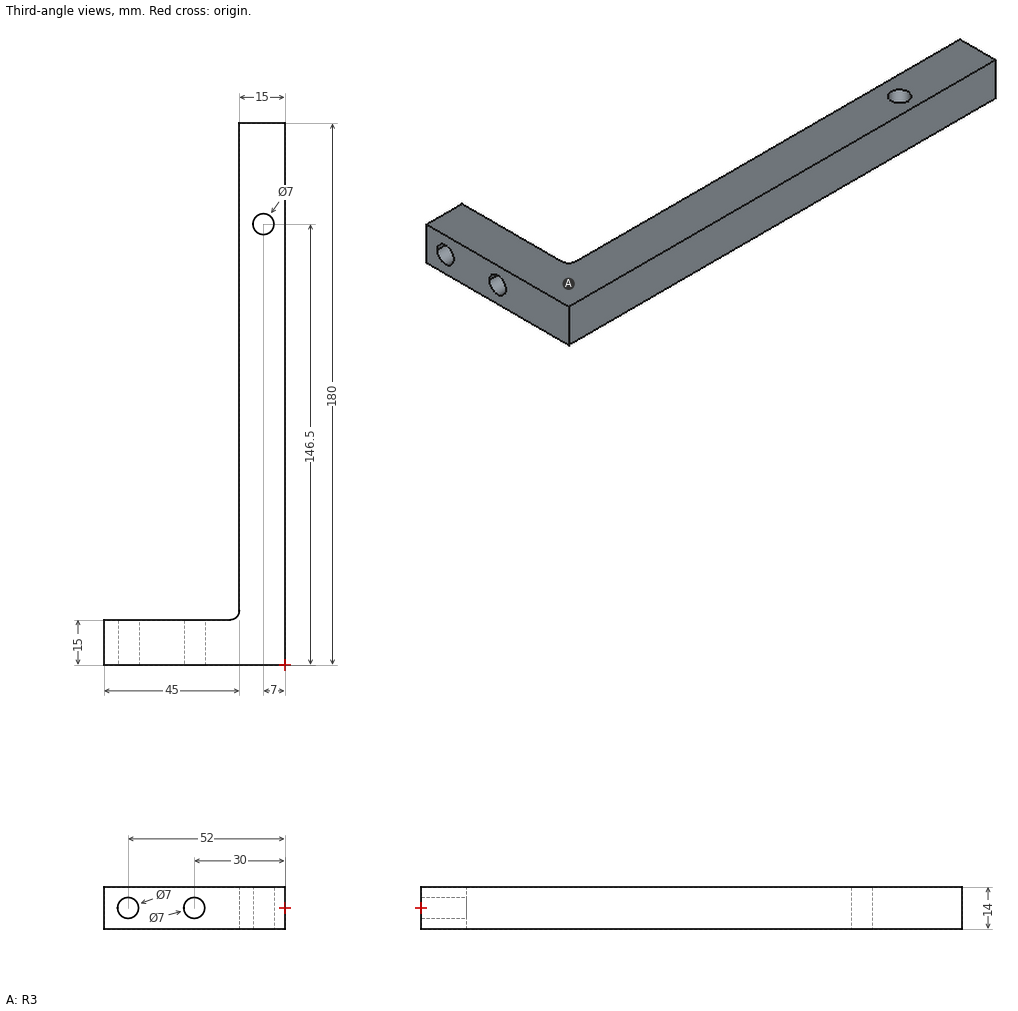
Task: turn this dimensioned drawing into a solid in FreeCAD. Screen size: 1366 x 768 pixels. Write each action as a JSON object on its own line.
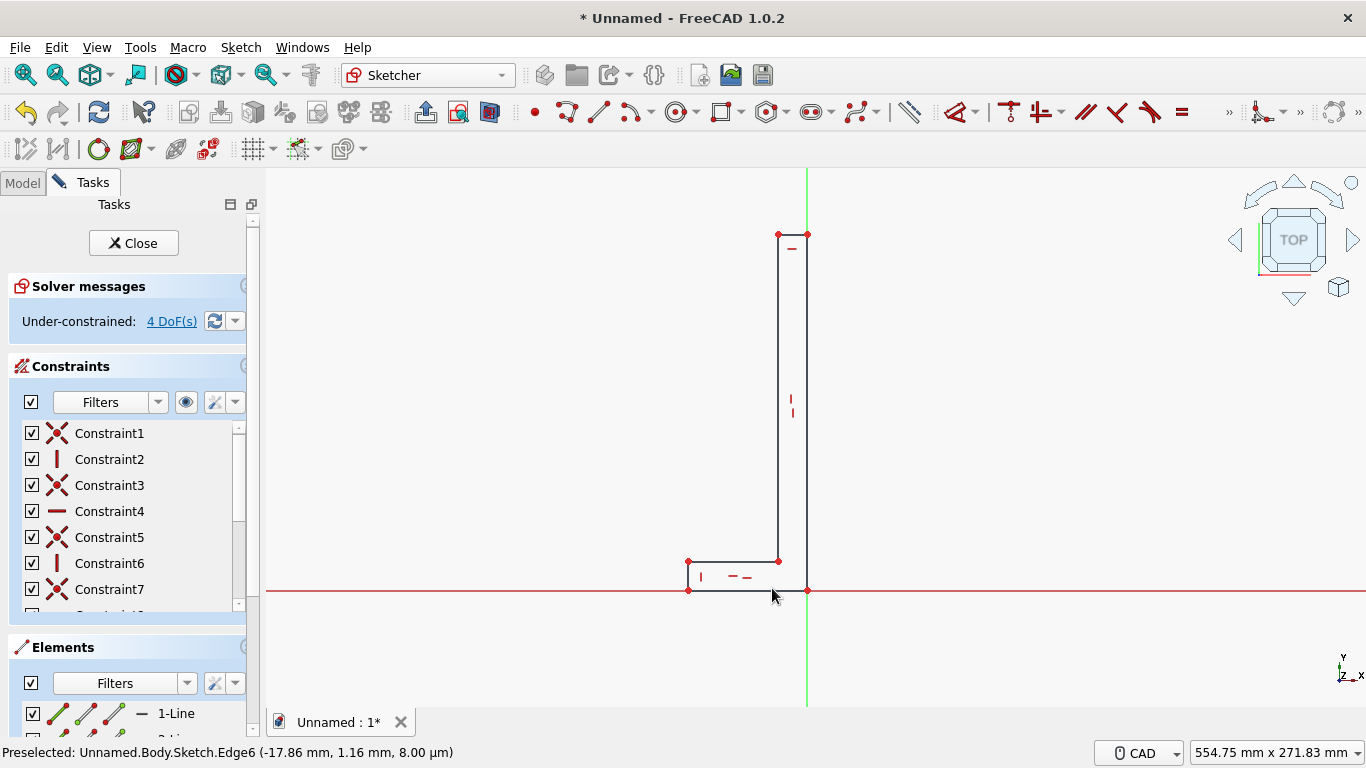
{"action": "left_click", "coordinate": [956, 112]}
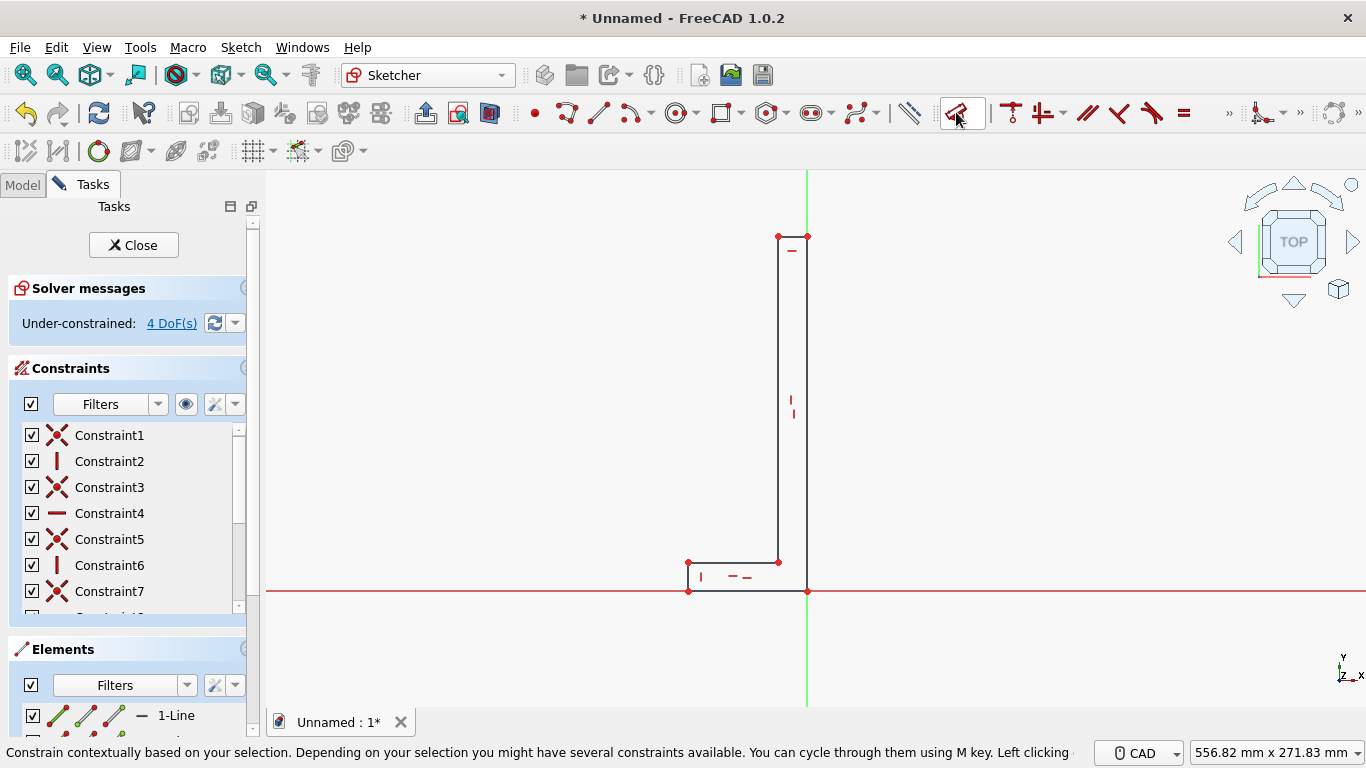
{"action": "scroll", "coordinate": [796, 237], "scroll_direction": "up", "scroll_amount": 2}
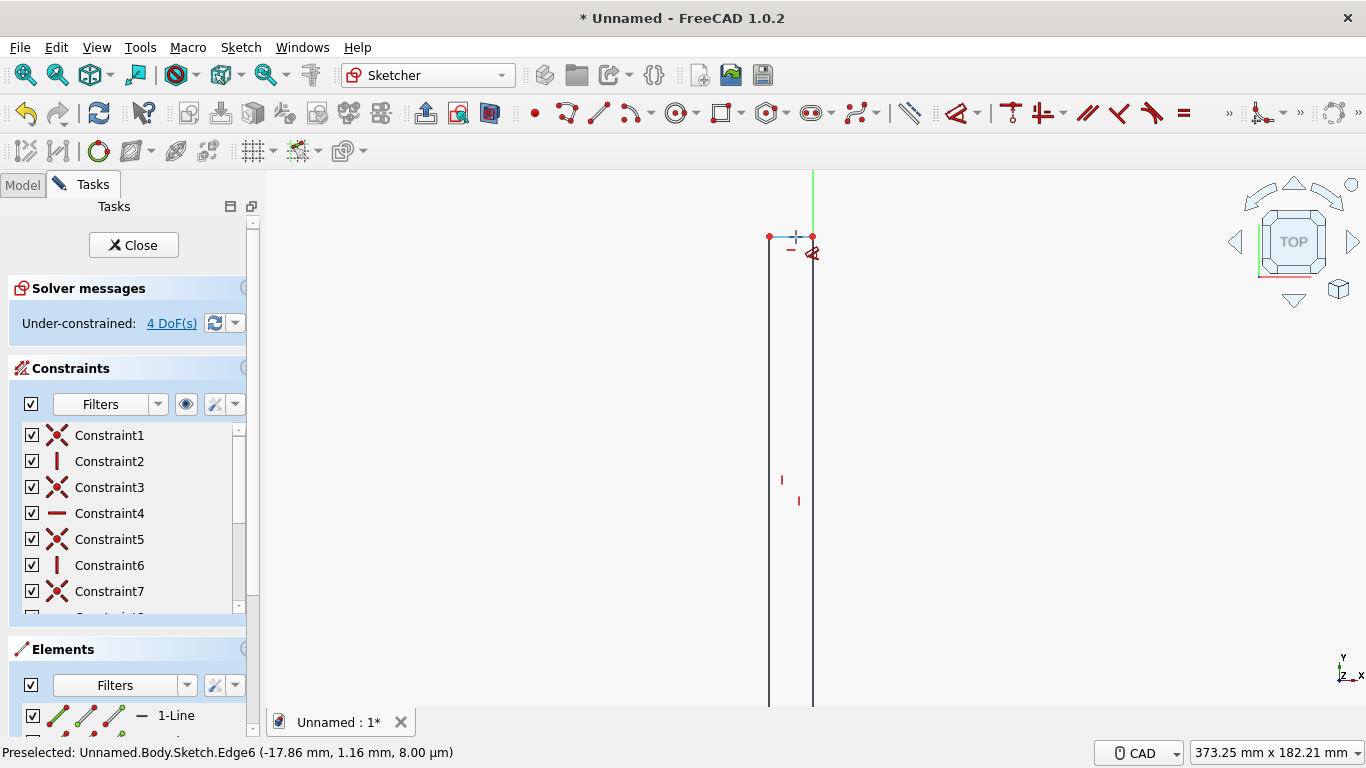
{"action": "left_click", "coordinate": [795, 237]}
{"action": "left_click", "coordinate": [791, 203]}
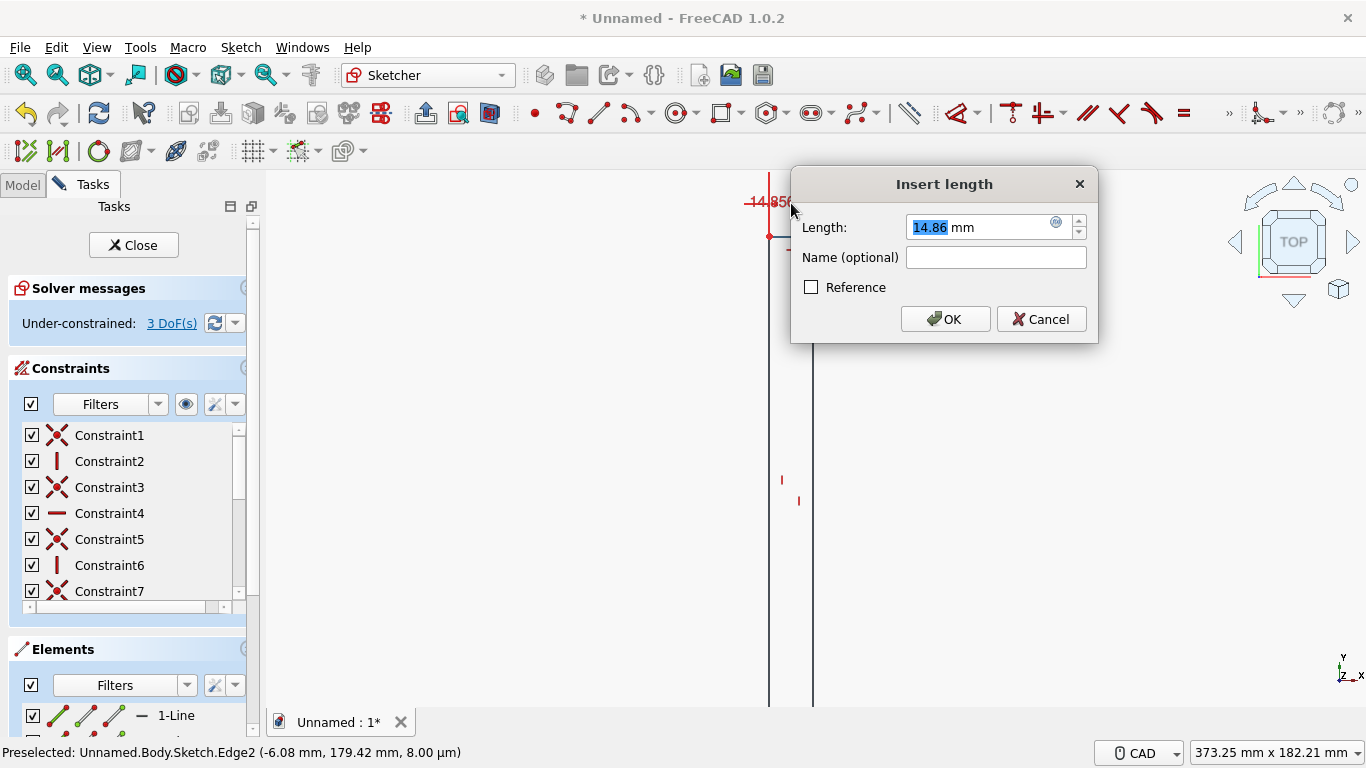
{"action": "type", "text": "15"}
{"action": "key", "text": "Return"}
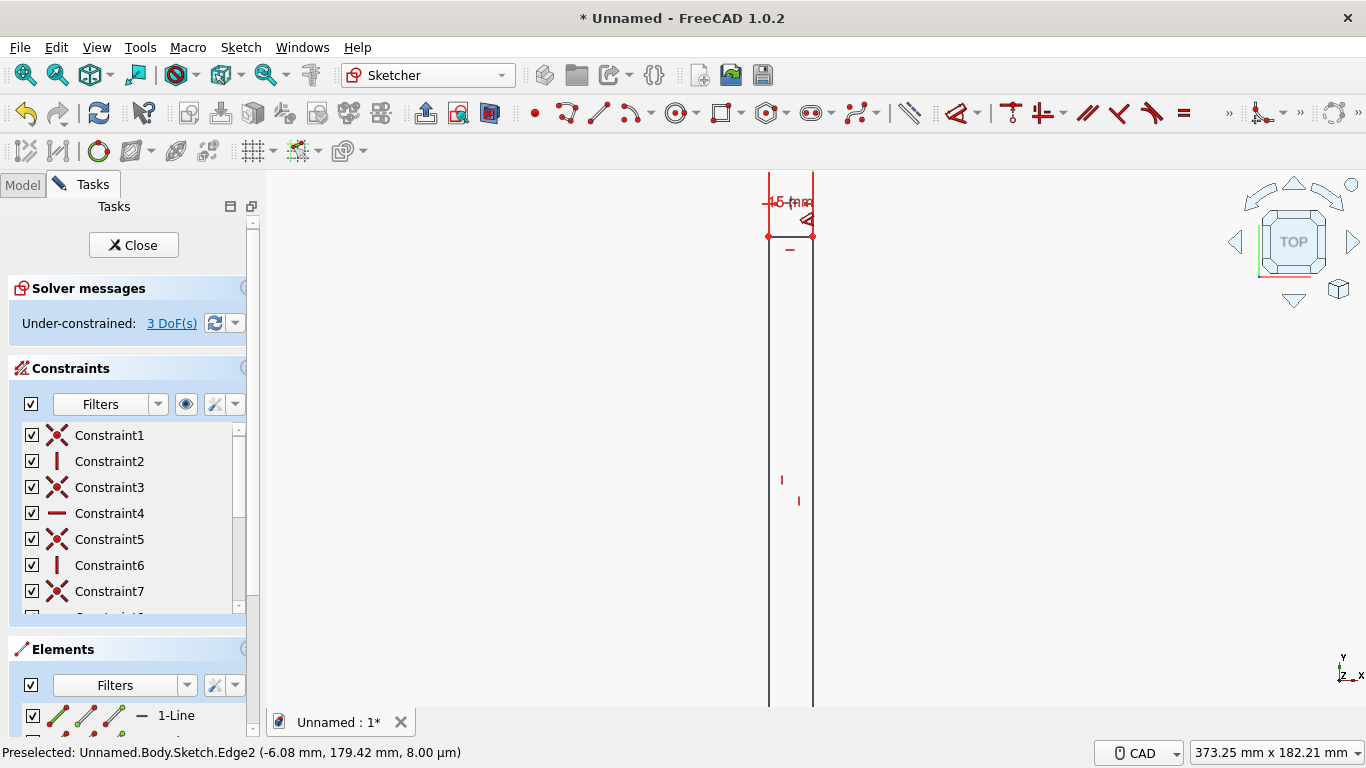
{"action": "scroll", "coordinate": [794, 313], "scroll_direction": "down", "scroll_amount": 2}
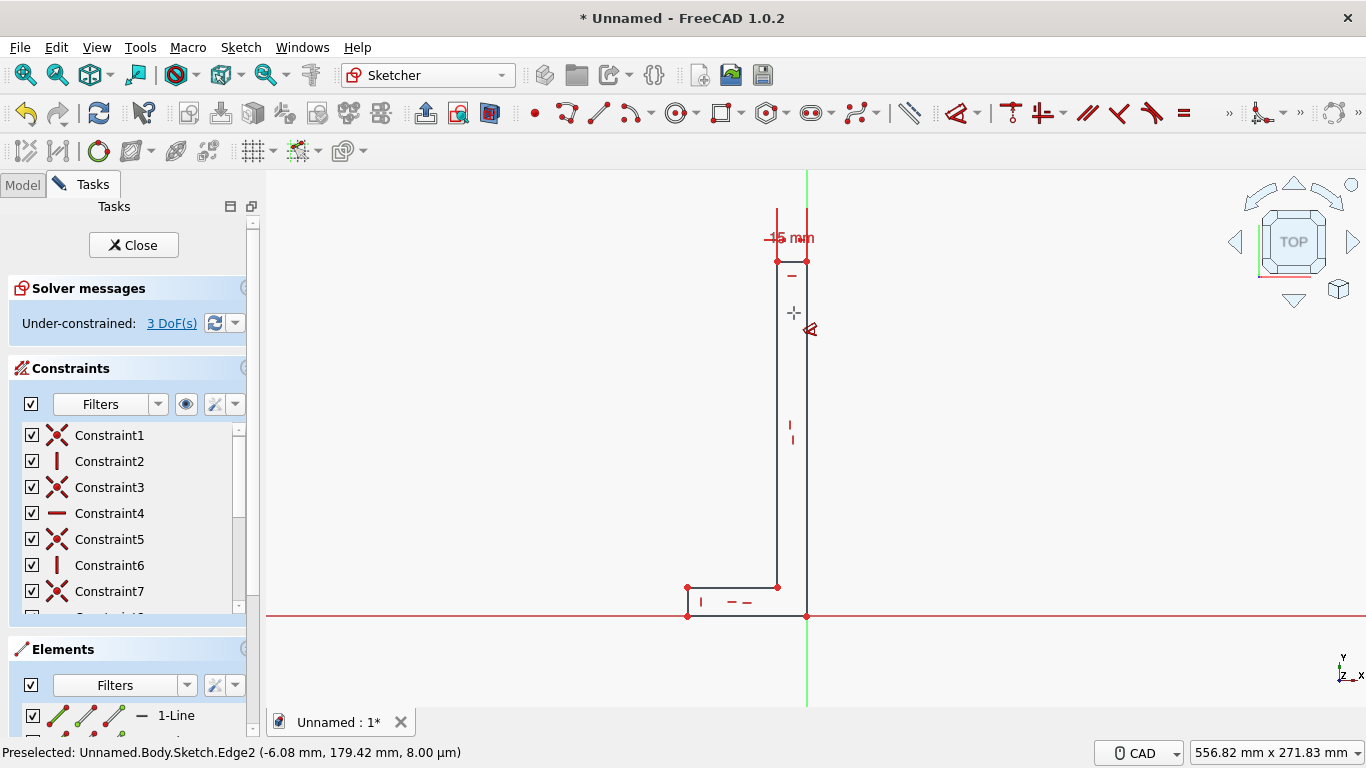
{"action": "left_click", "coordinate": [750, 588]}
{"action": "left_click", "coordinate": [733, 554]}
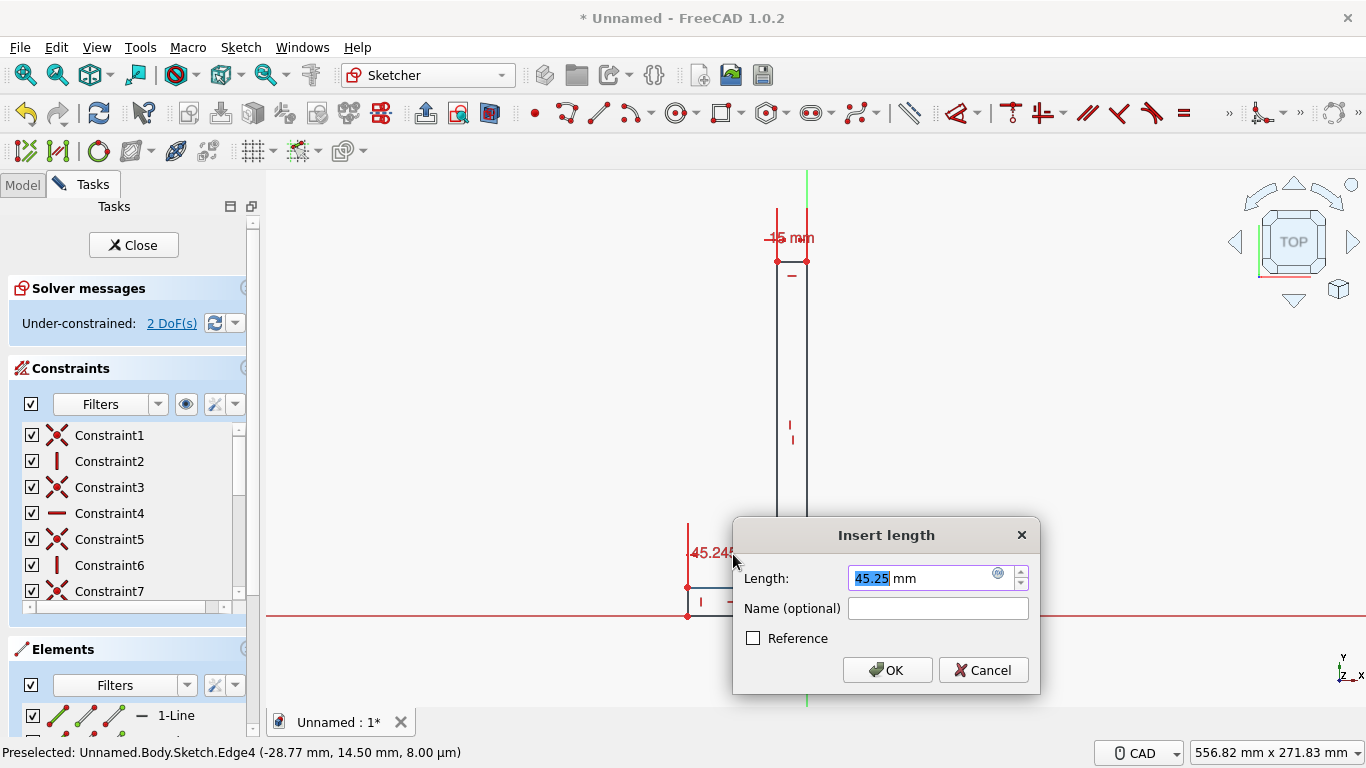
{"action": "type", "text": "45"}
{"action": "key", "text": "Return"}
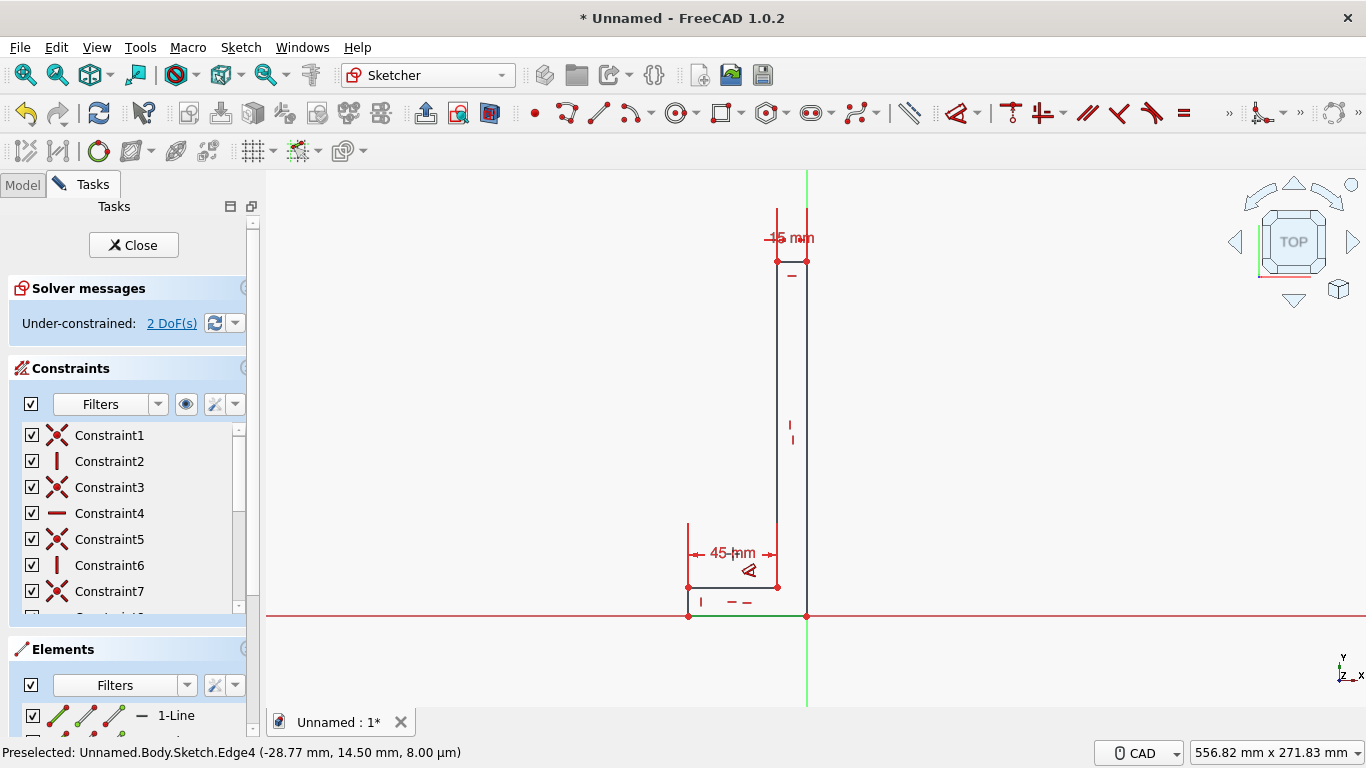
{"action": "scroll", "coordinate": [688, 599], "scroll_direction": "up", "scroll_amount": 2}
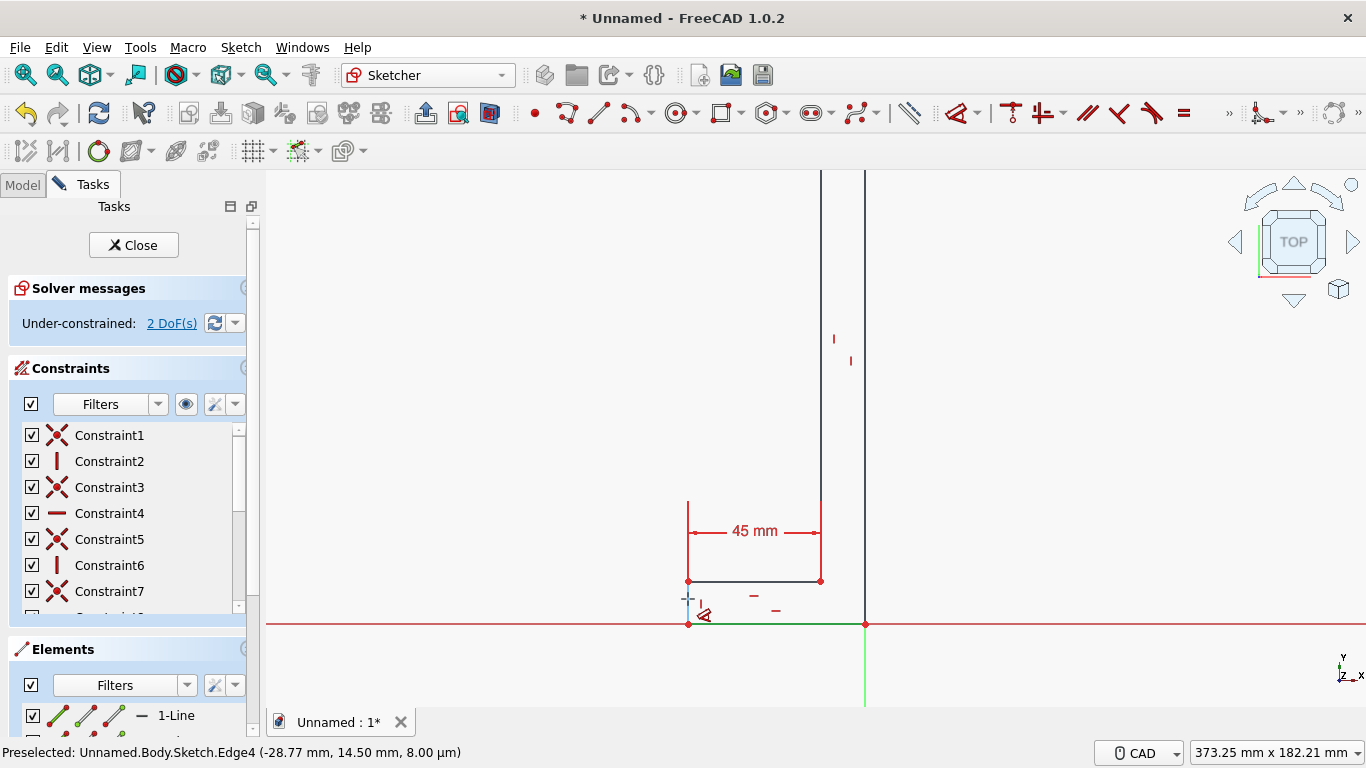
{"action": "left_click", "coordinate": [688, 599]}
{"action": "left_click", "coordinate": [654, 603]}